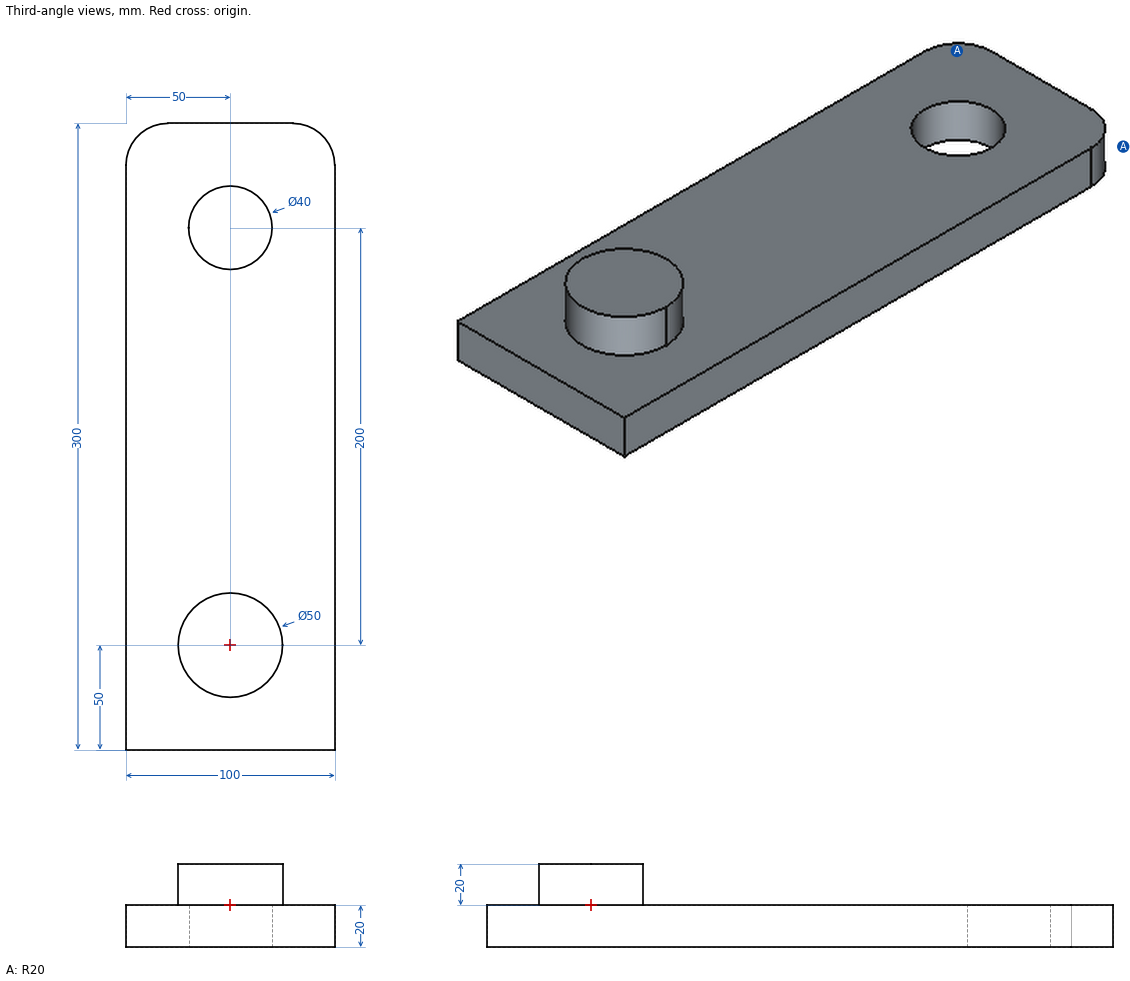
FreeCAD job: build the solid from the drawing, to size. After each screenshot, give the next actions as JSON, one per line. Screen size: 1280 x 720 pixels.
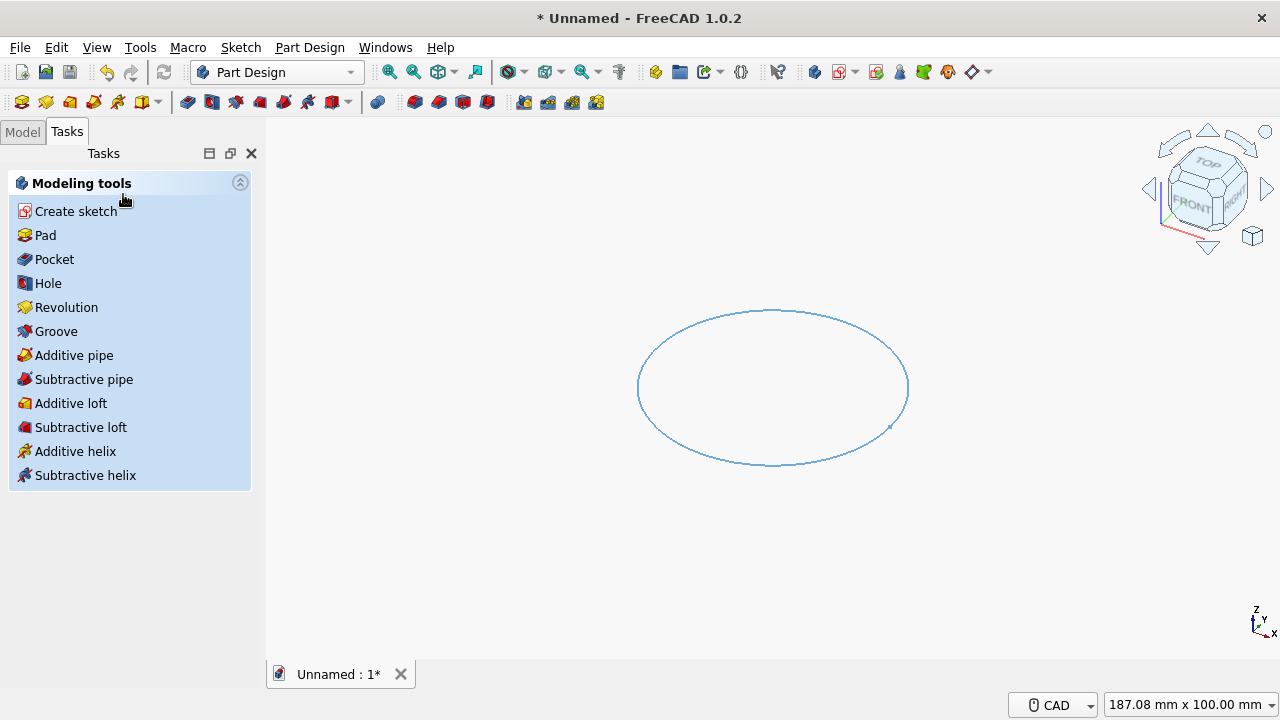
{"action": "left_click", "coordinate": [22, 102]}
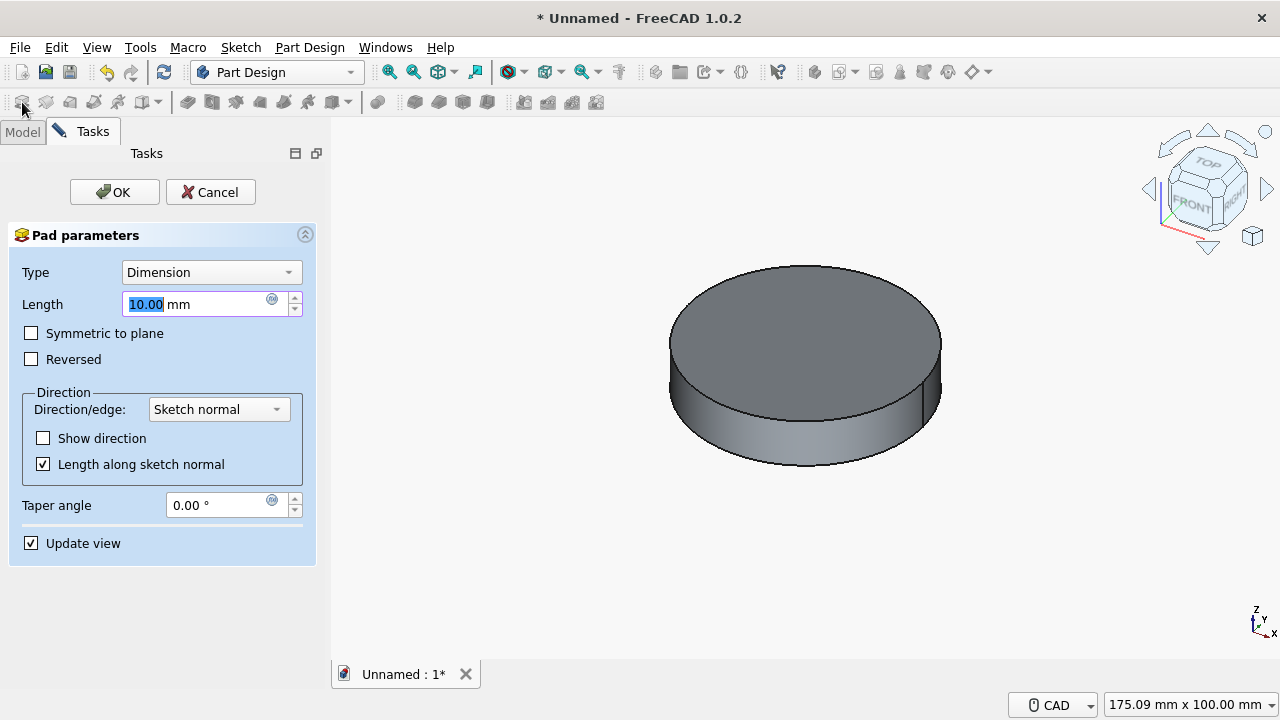
{"action": "type", "text": "20"}
{"action": "key", "text": "Tab"}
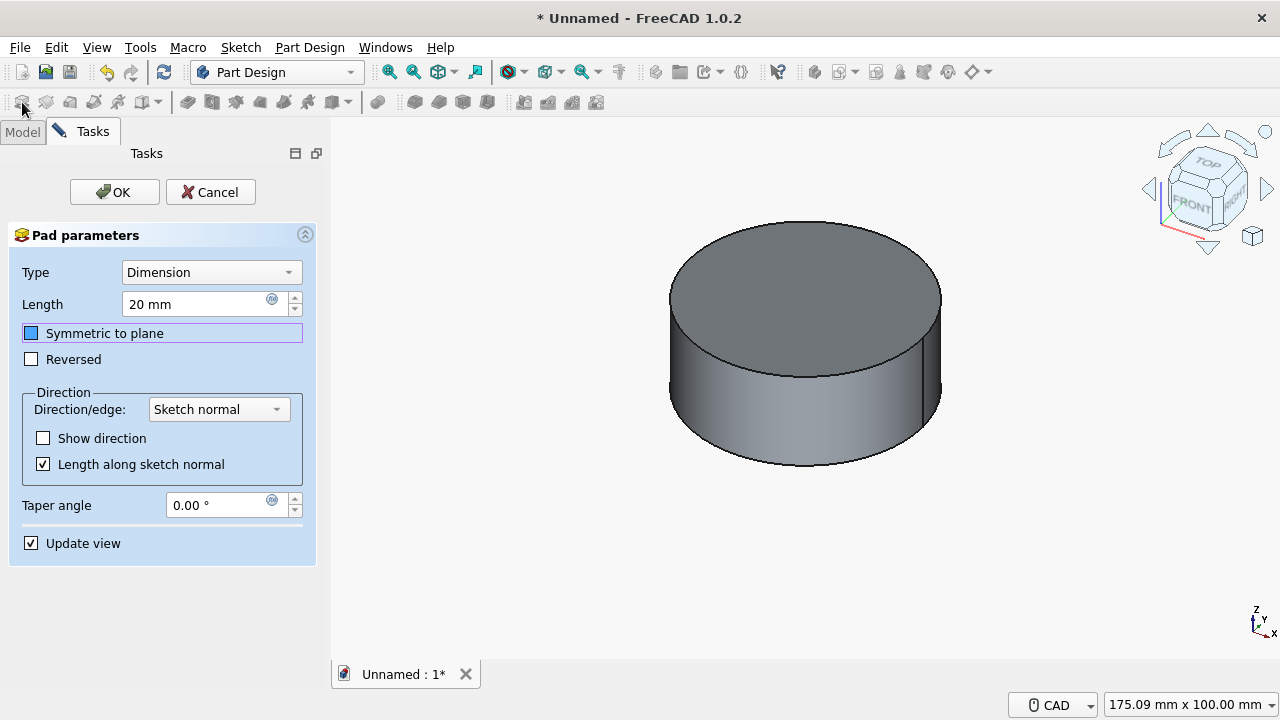
{"action": "left_click", "coordinate": [115, 192]}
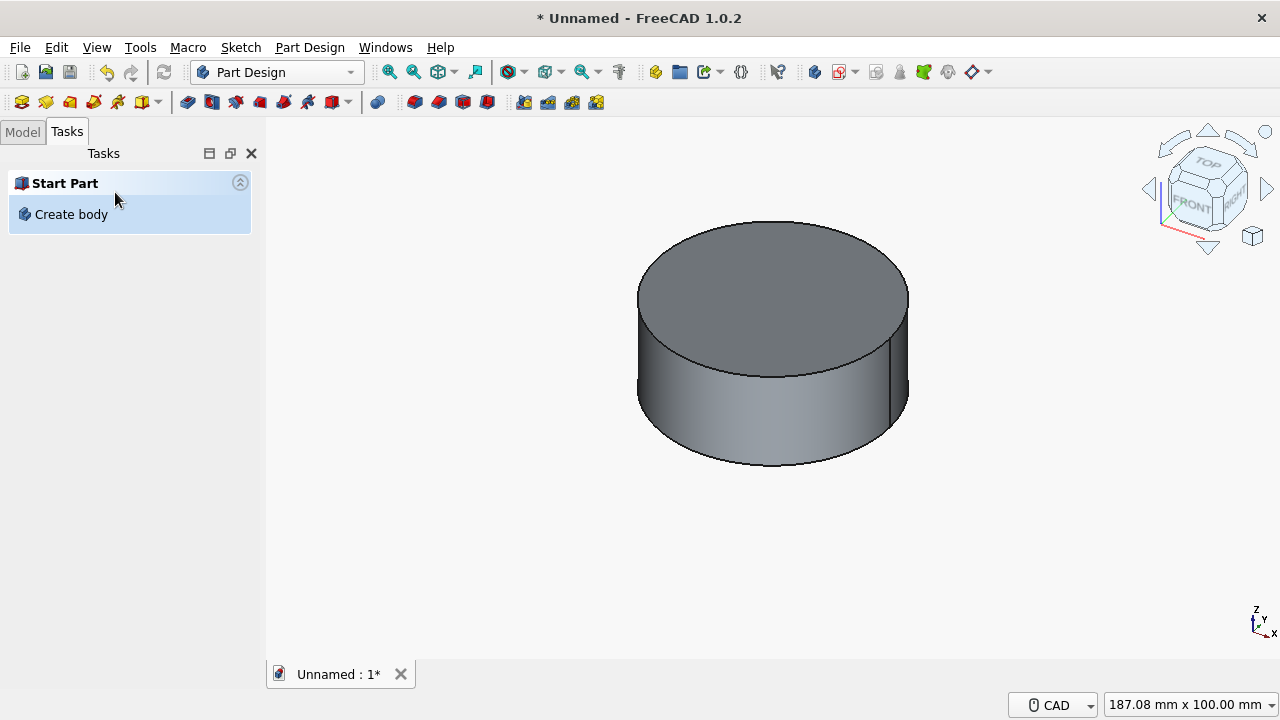
{"action": "left_click", "coordinate": [840, 72]}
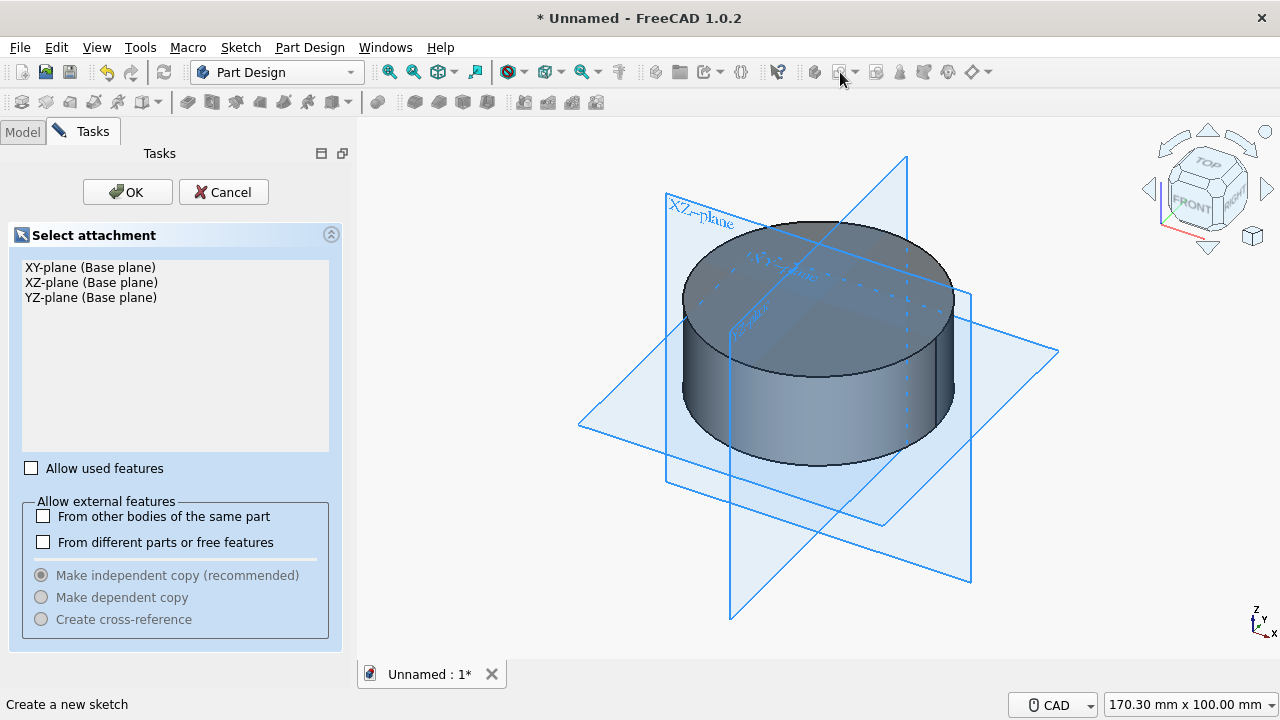
{"action": "left_click", "coordinate": [82, 268]}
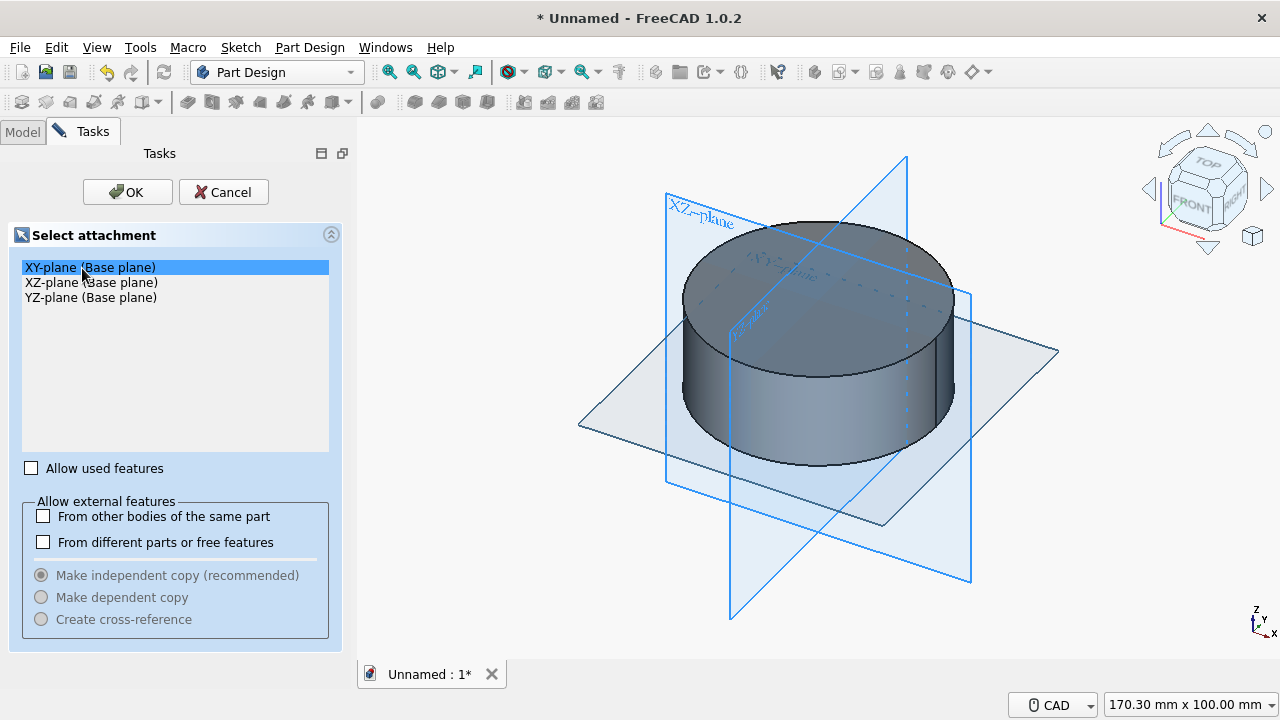
{"action": "left_click", "coordinate": [128, 192]}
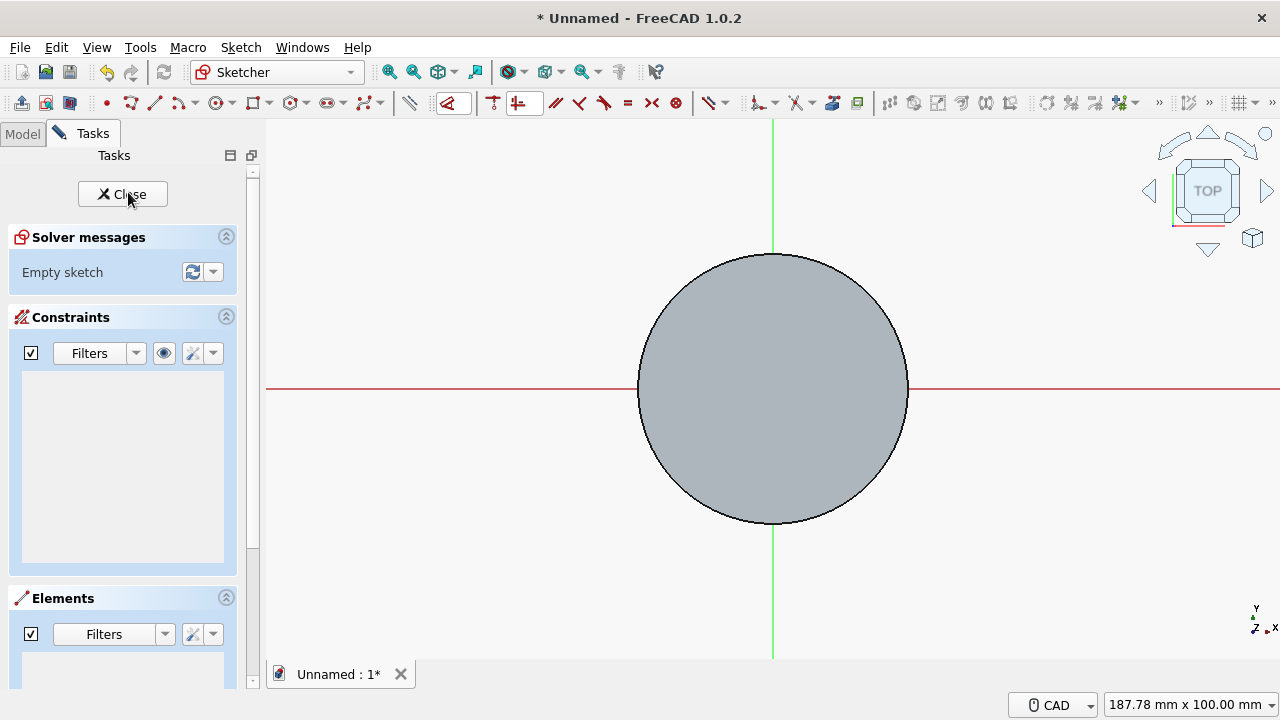
{"action": "left_click", "coordinate": [70, 104]}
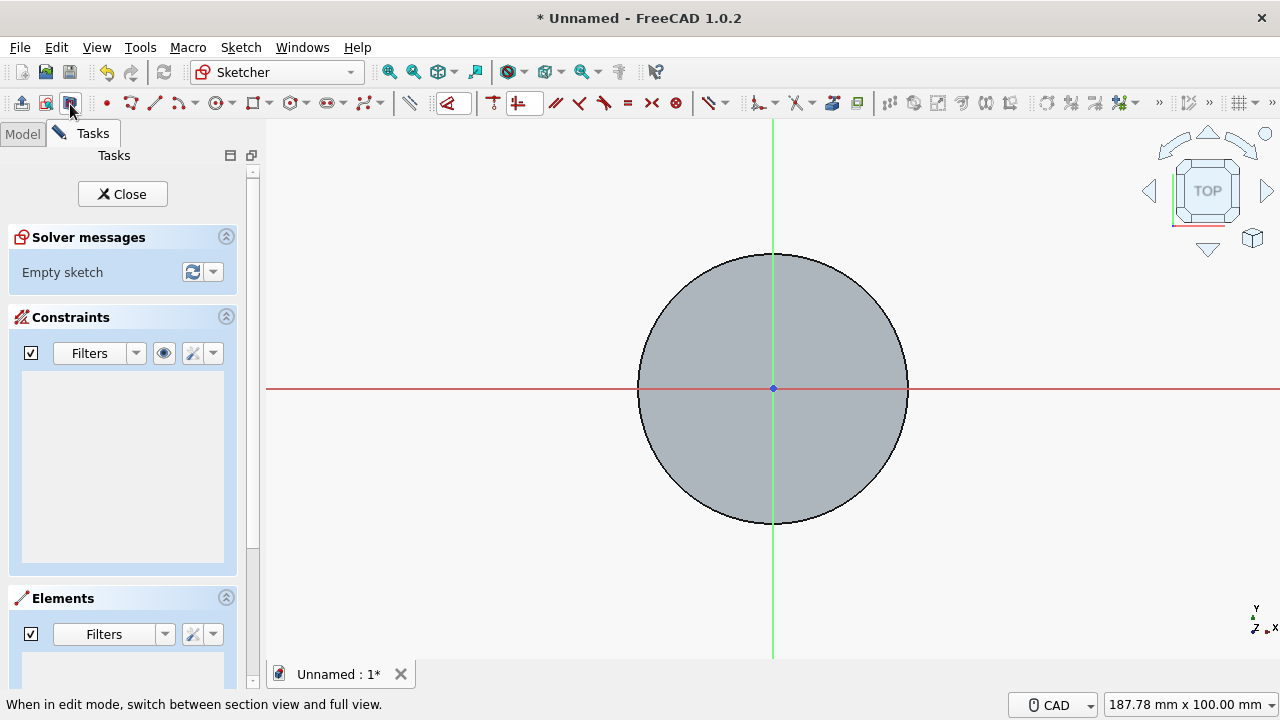
{"action": "scroll", "coordinate": [687, 526], "scroll_direction": "down", "scroll_amount": 8}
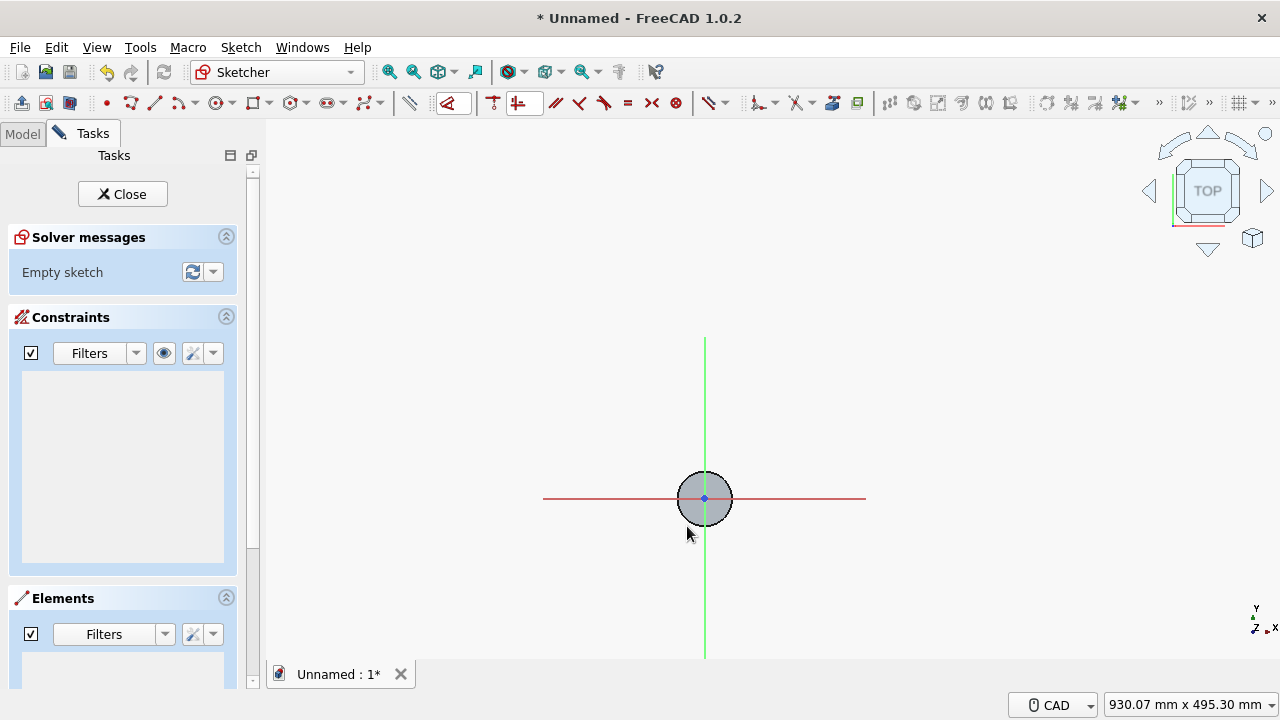
{"action": "left_click", "coordinate": [254, 104]}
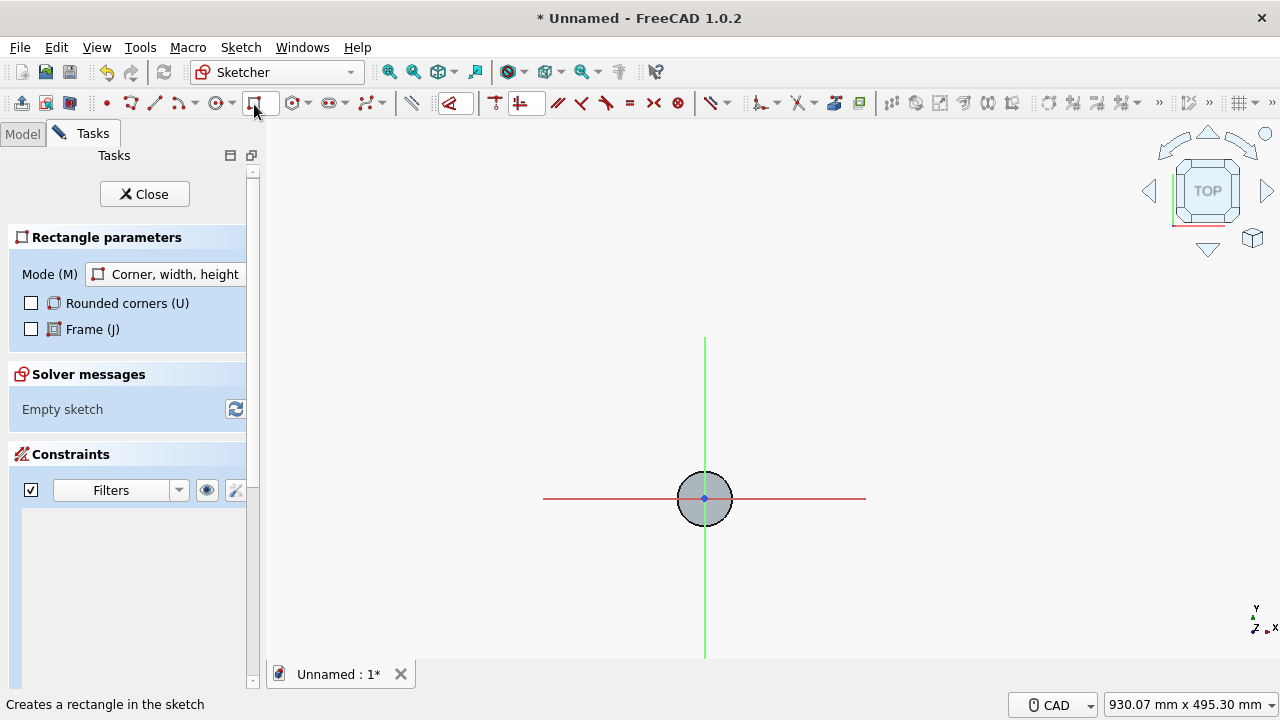
{"action": "left_click", "coordinate": [650, 226]}
{"action": "left_click", "coordinate": [759, 553]}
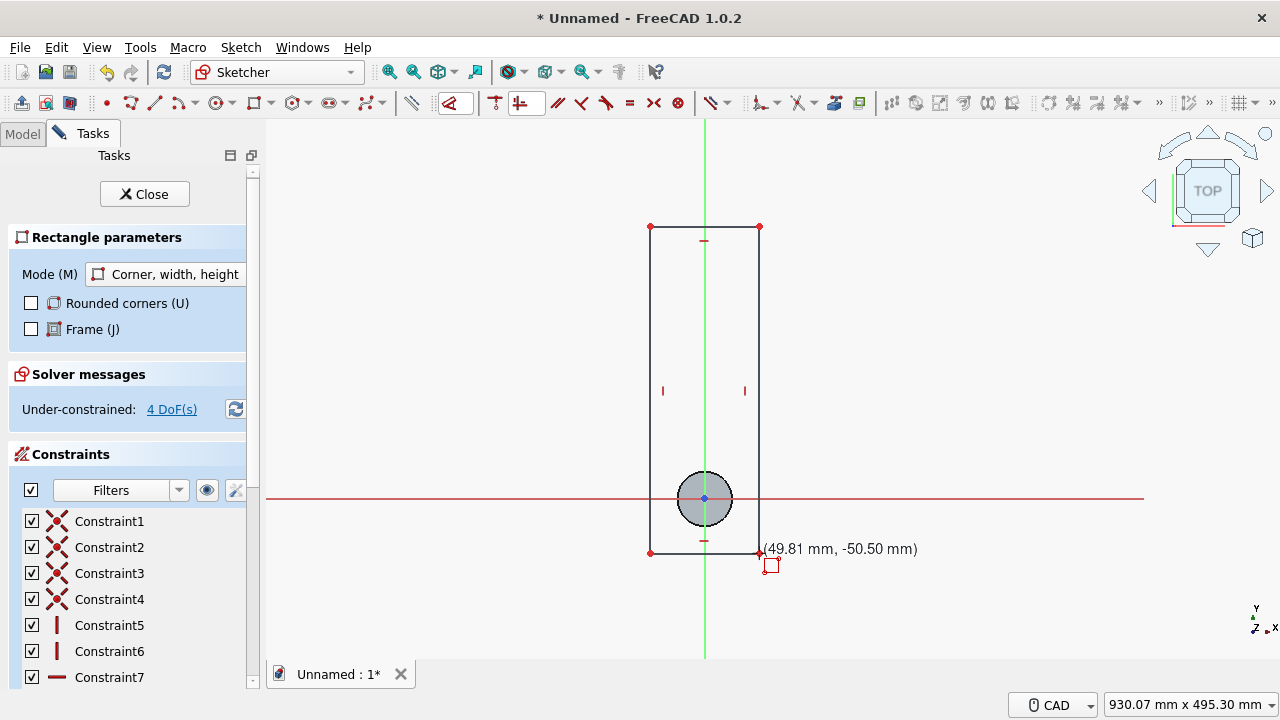
{"action": "left_click", "coordinate": [216, 104]}